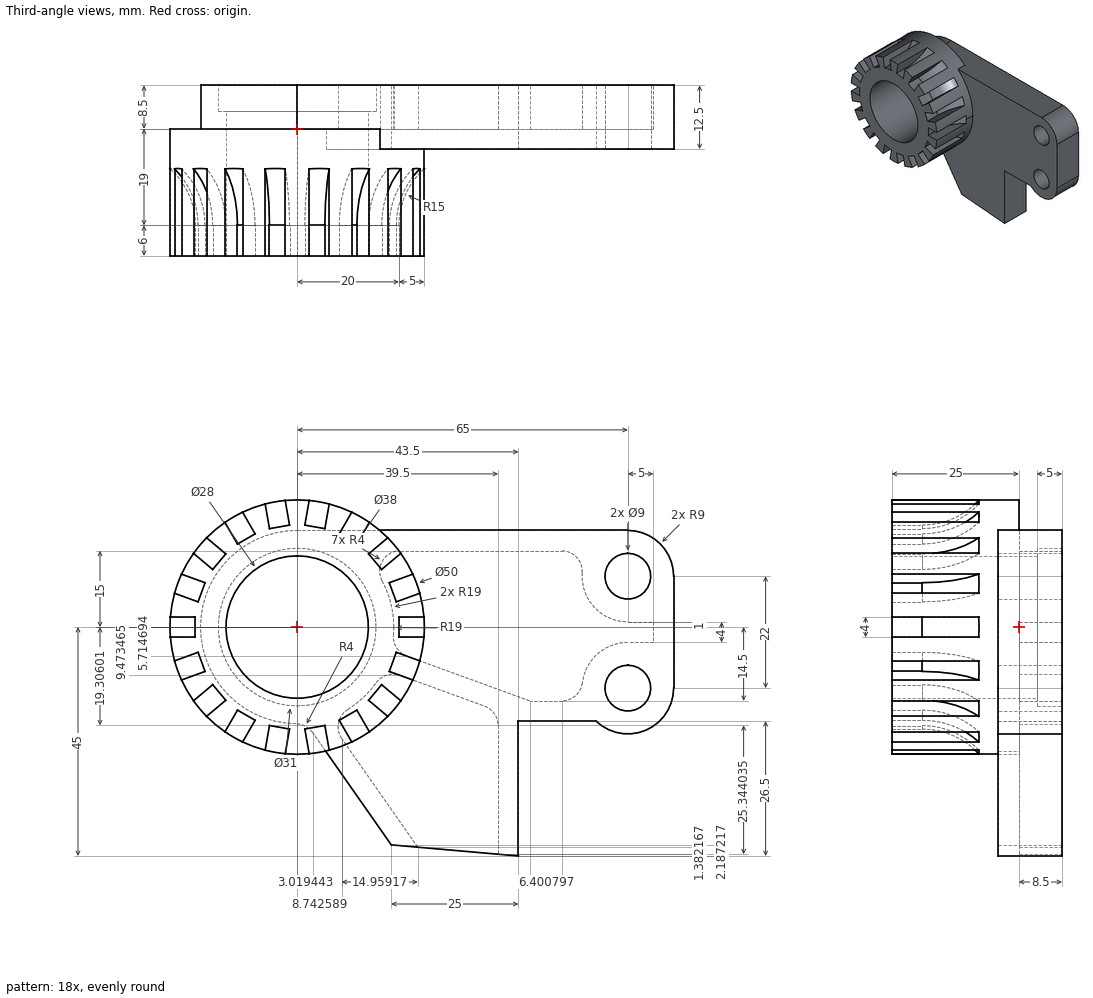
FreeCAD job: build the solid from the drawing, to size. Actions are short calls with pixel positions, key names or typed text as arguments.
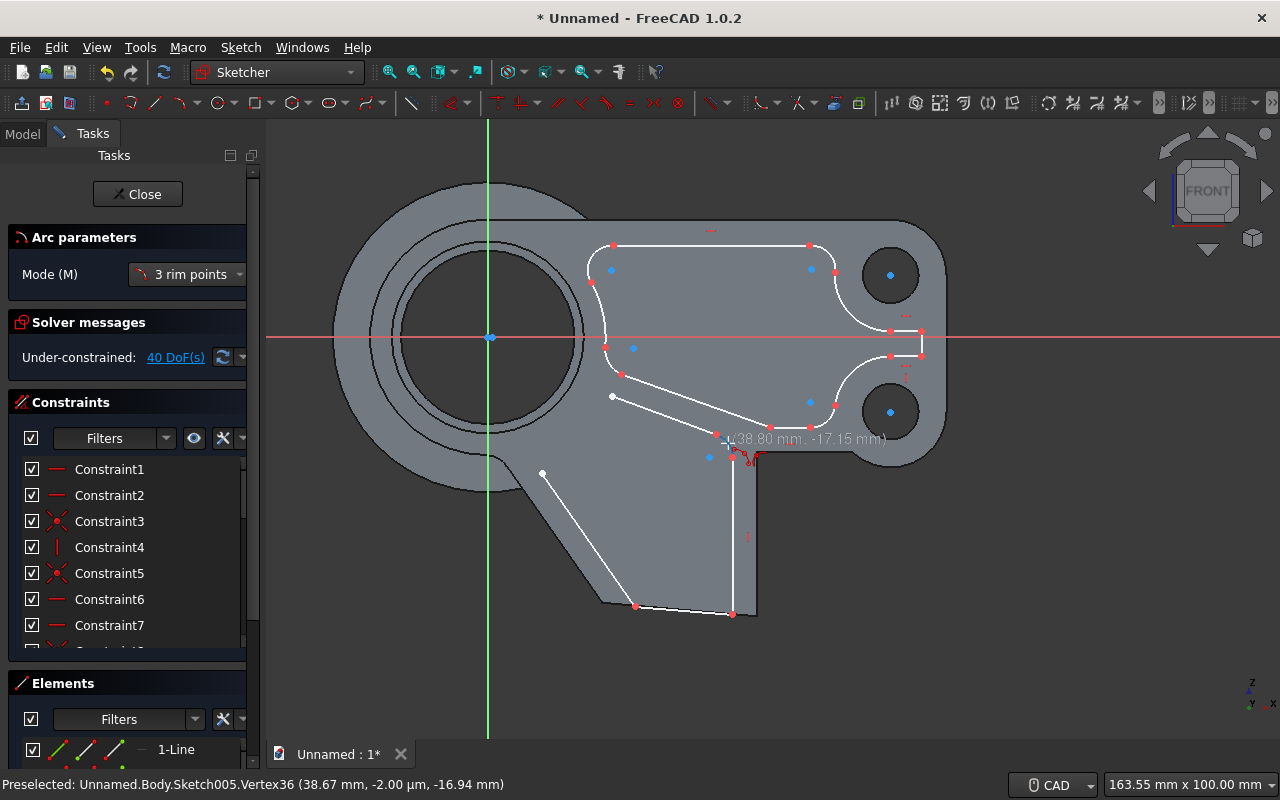
click(542, 474)
click(549, 438)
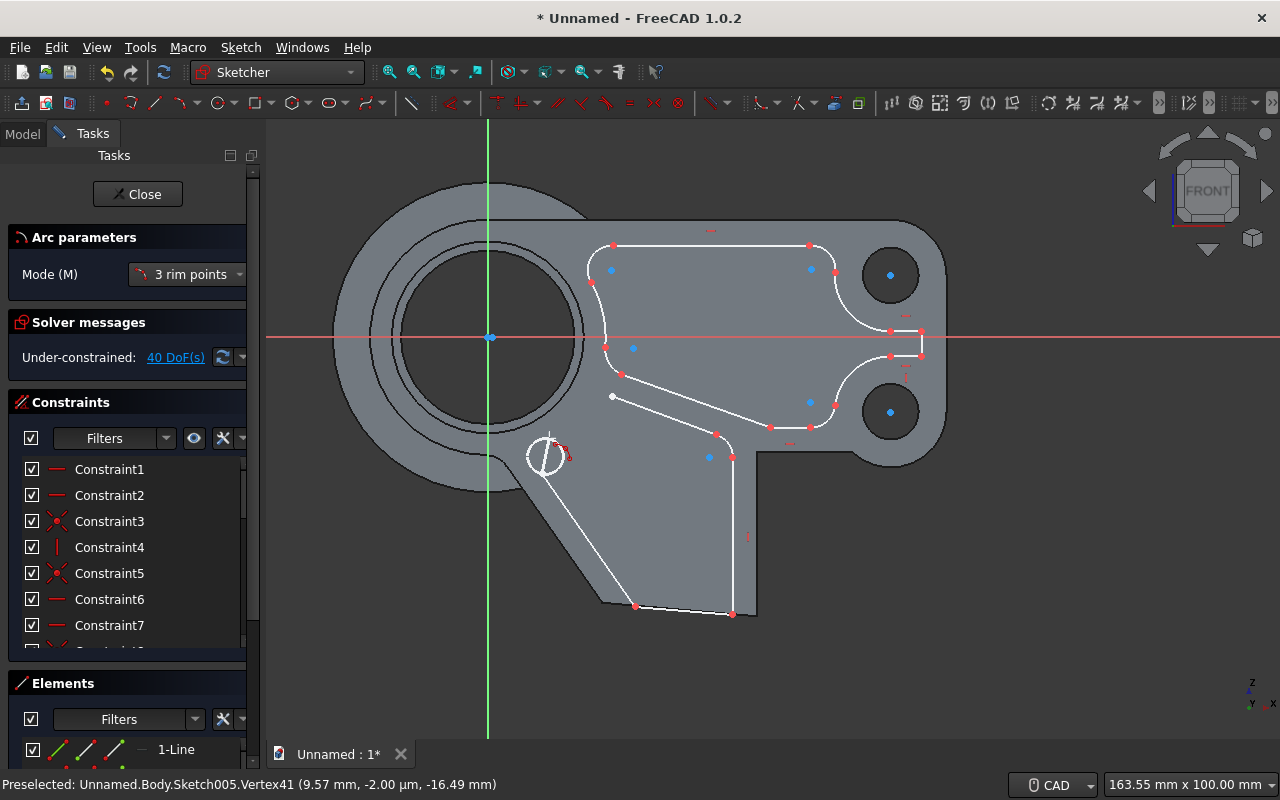
scroll(538, 454, up, 4)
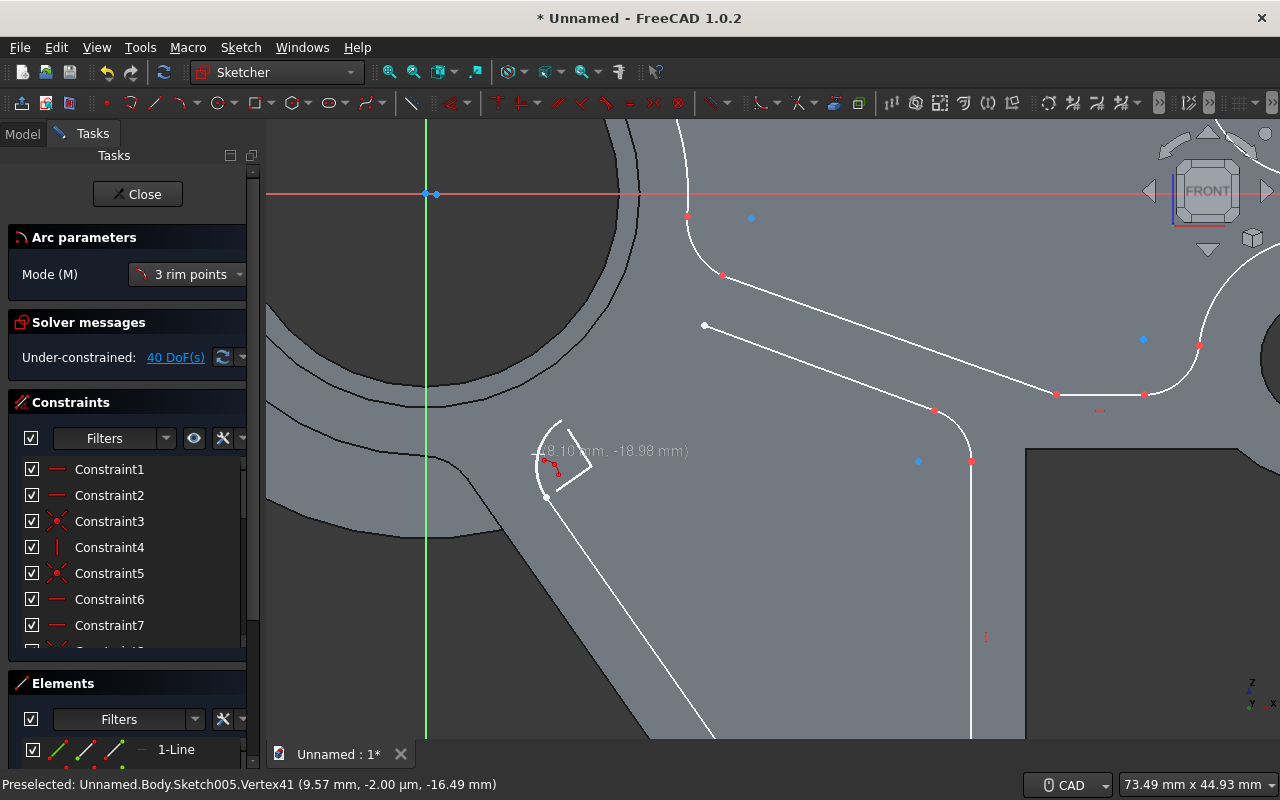
click(538, 453)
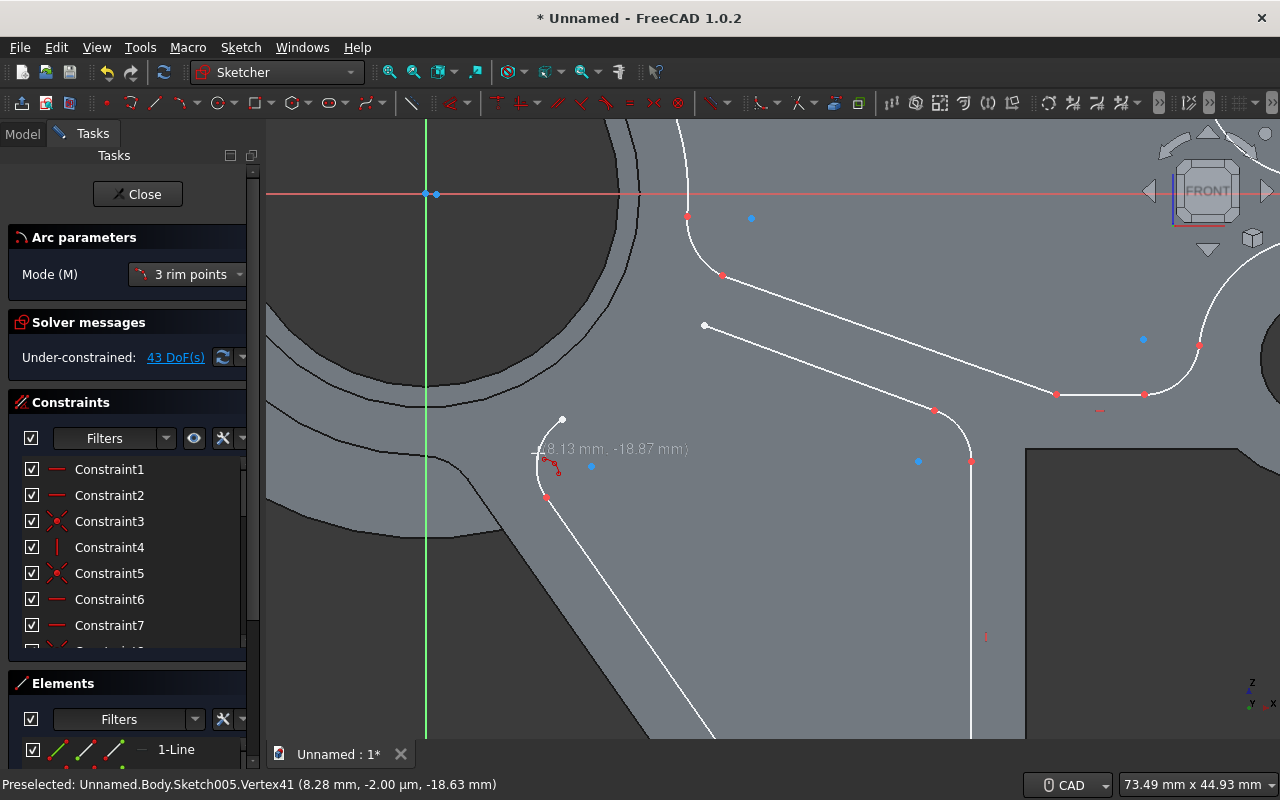
click(562, 420)
click(640, 344)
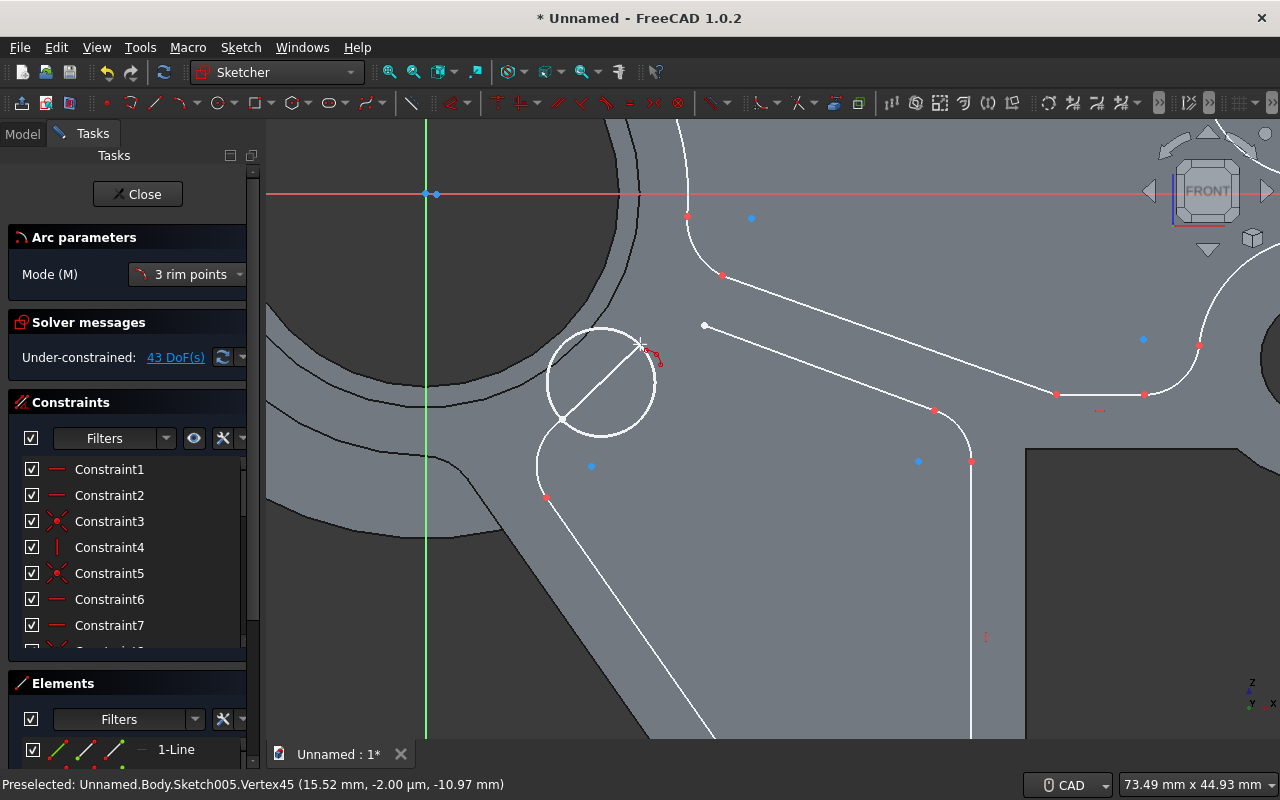
scroll(605, 385, up, 6)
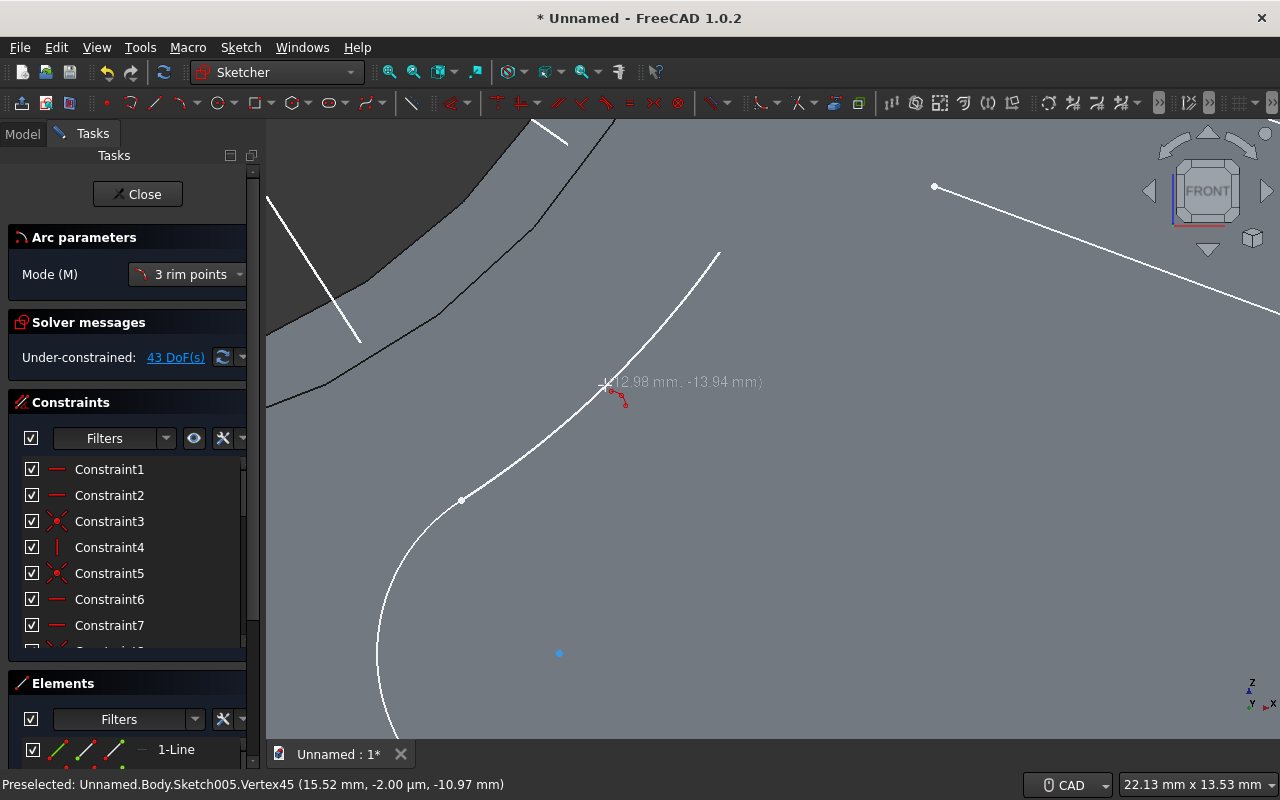
click(605, 383)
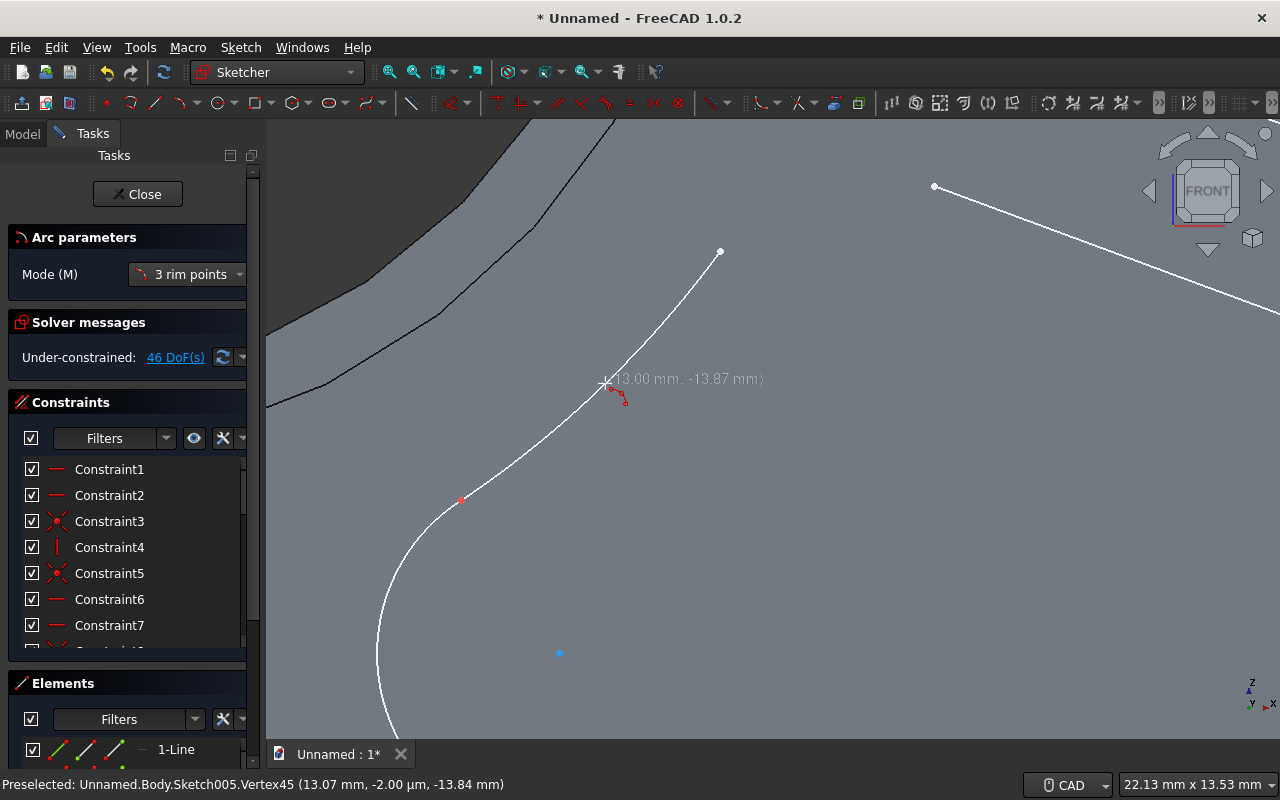
scroll(562, 429, down, 10)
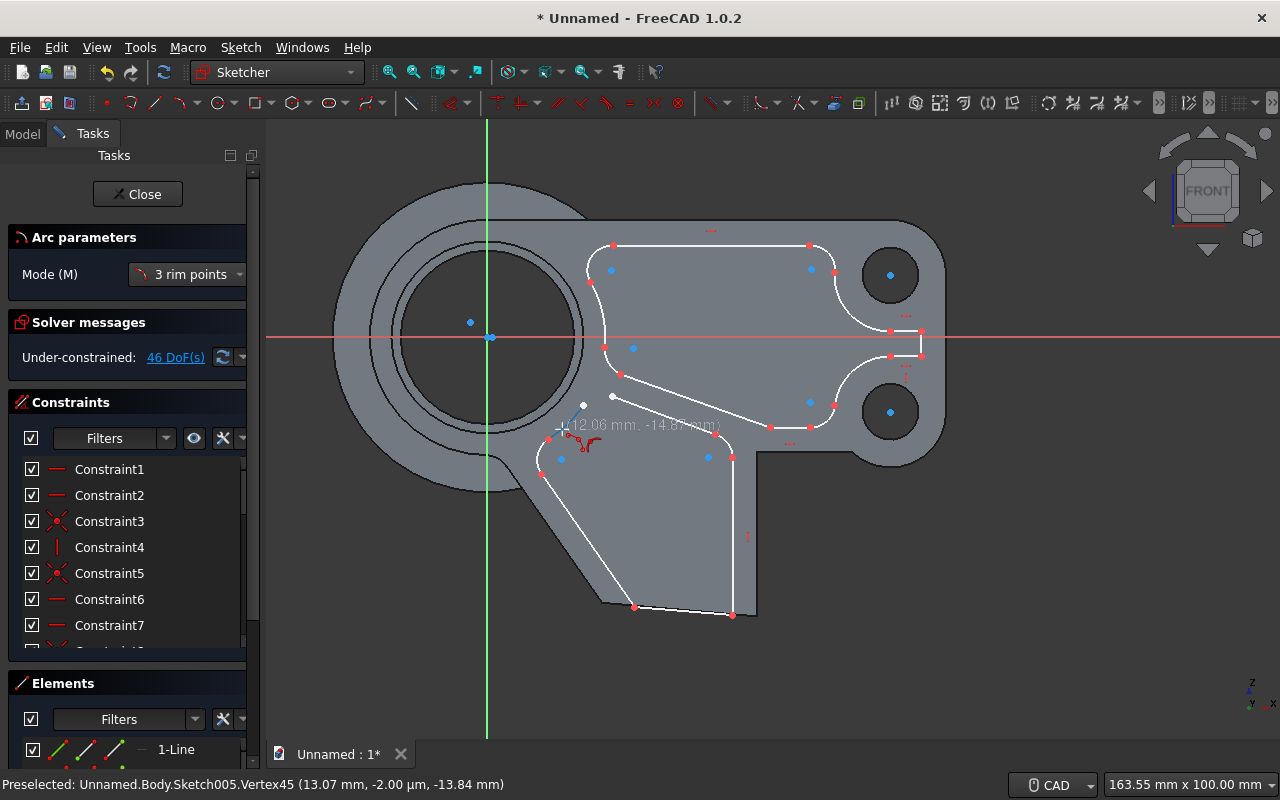
click(584, 405)
click(613, 397)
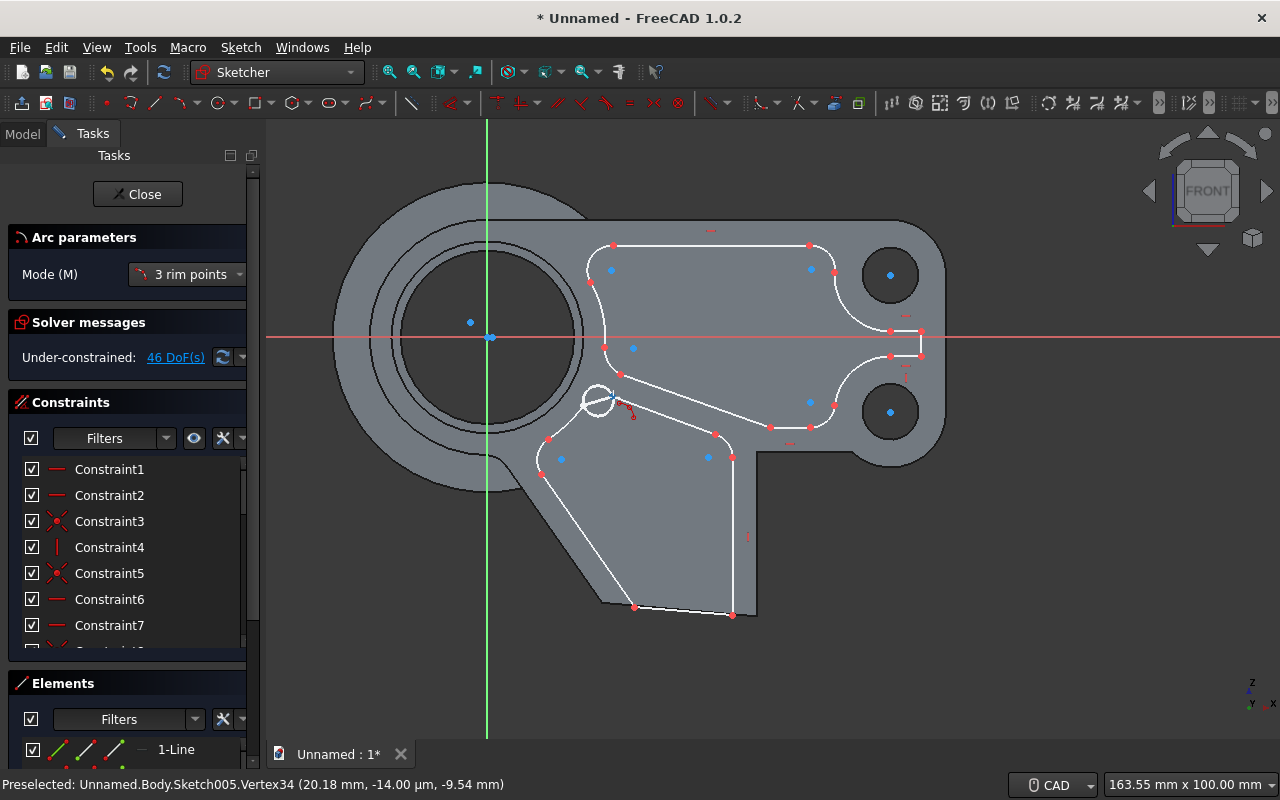
scroll(597, 396, up, 6)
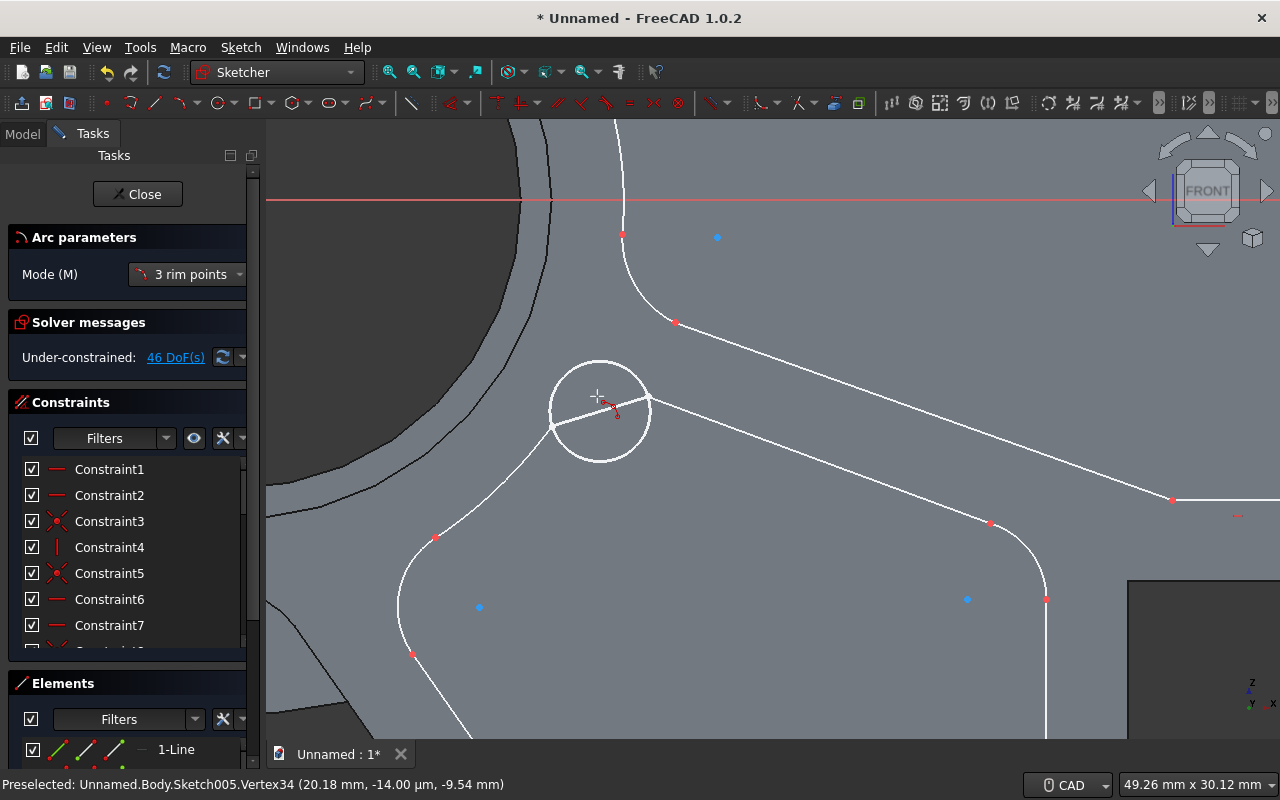
click(595, 394)
key(Escape)